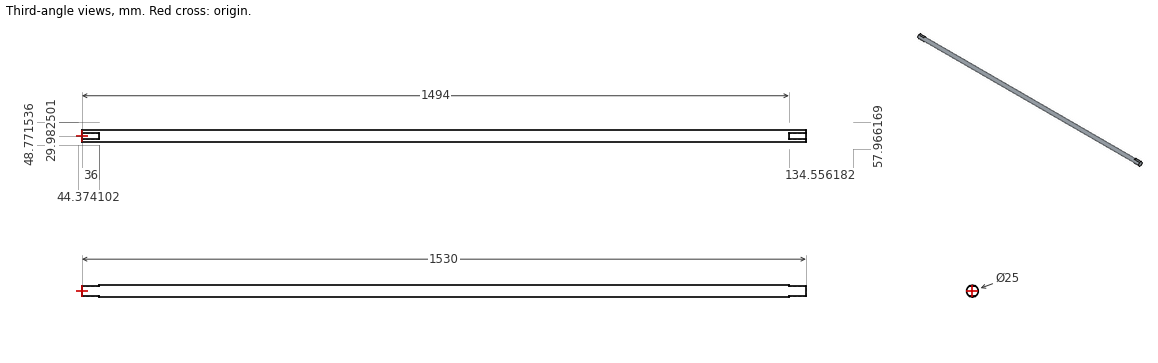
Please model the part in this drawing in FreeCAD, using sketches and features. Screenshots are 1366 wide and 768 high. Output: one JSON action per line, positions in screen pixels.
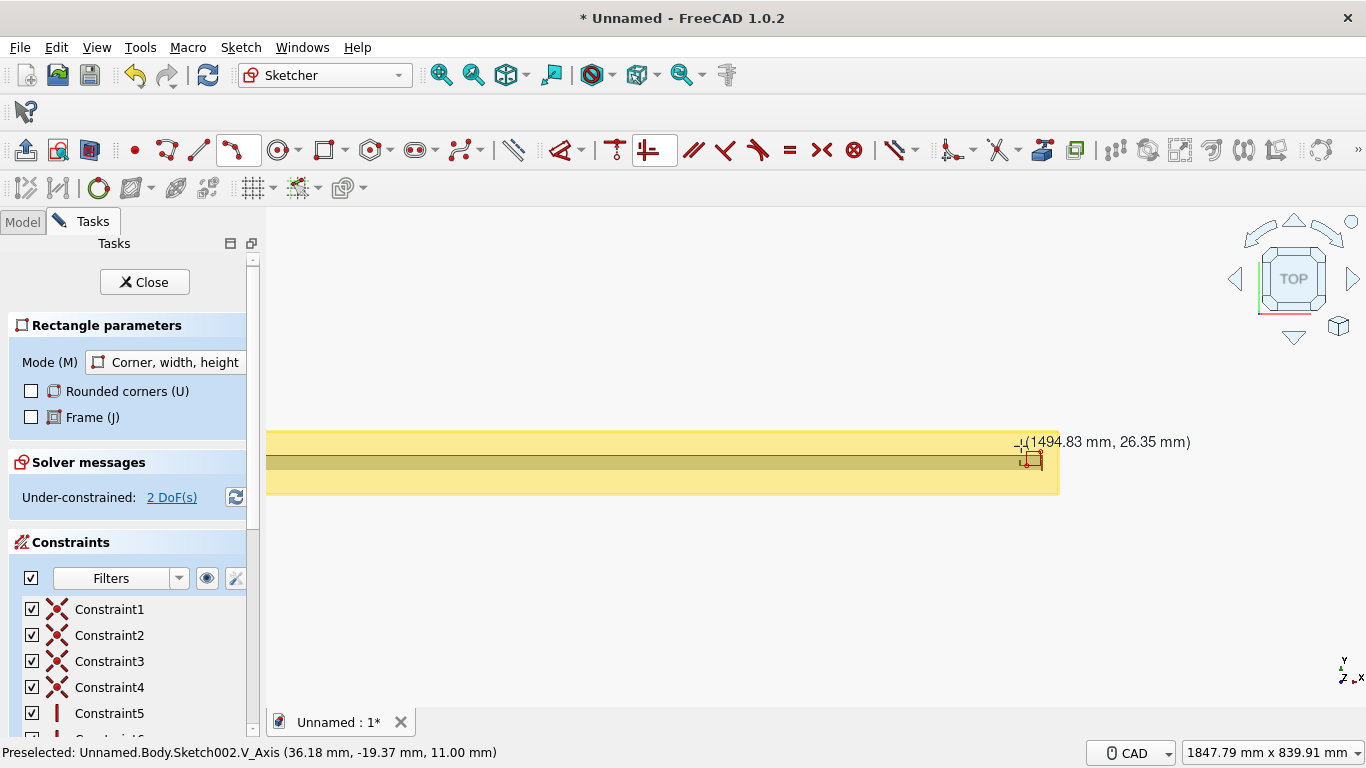
{"action": "left_click", "coordinate": [1020, 445]}
{"action": "mouse_move", "coordinate": [1100, 480]}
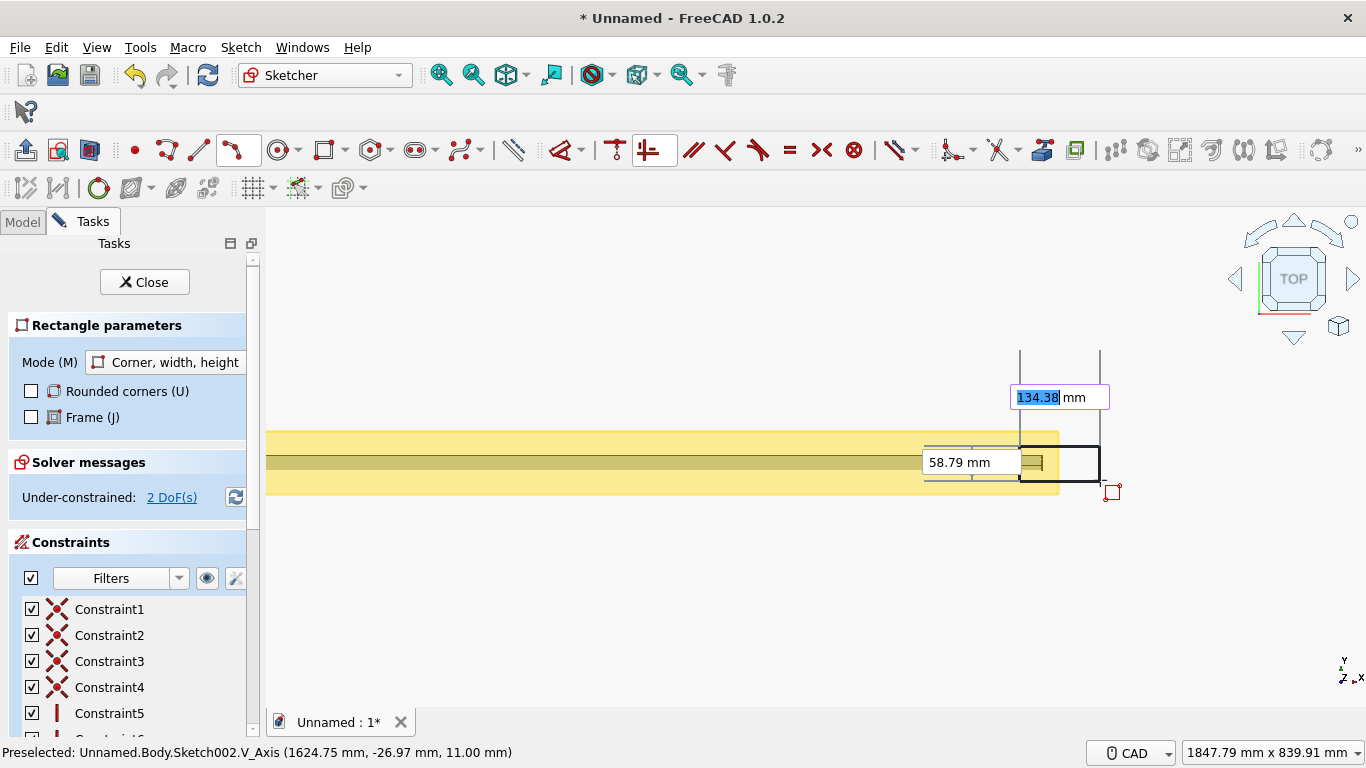
{"action": "type", "text": "134.556182"}
{"action": "key", "text": "Tab"}
{"action": "type", "text": "57.966169"}
{"action": "key", "text": "Return"}
{"action": "key", "text": "Escape"}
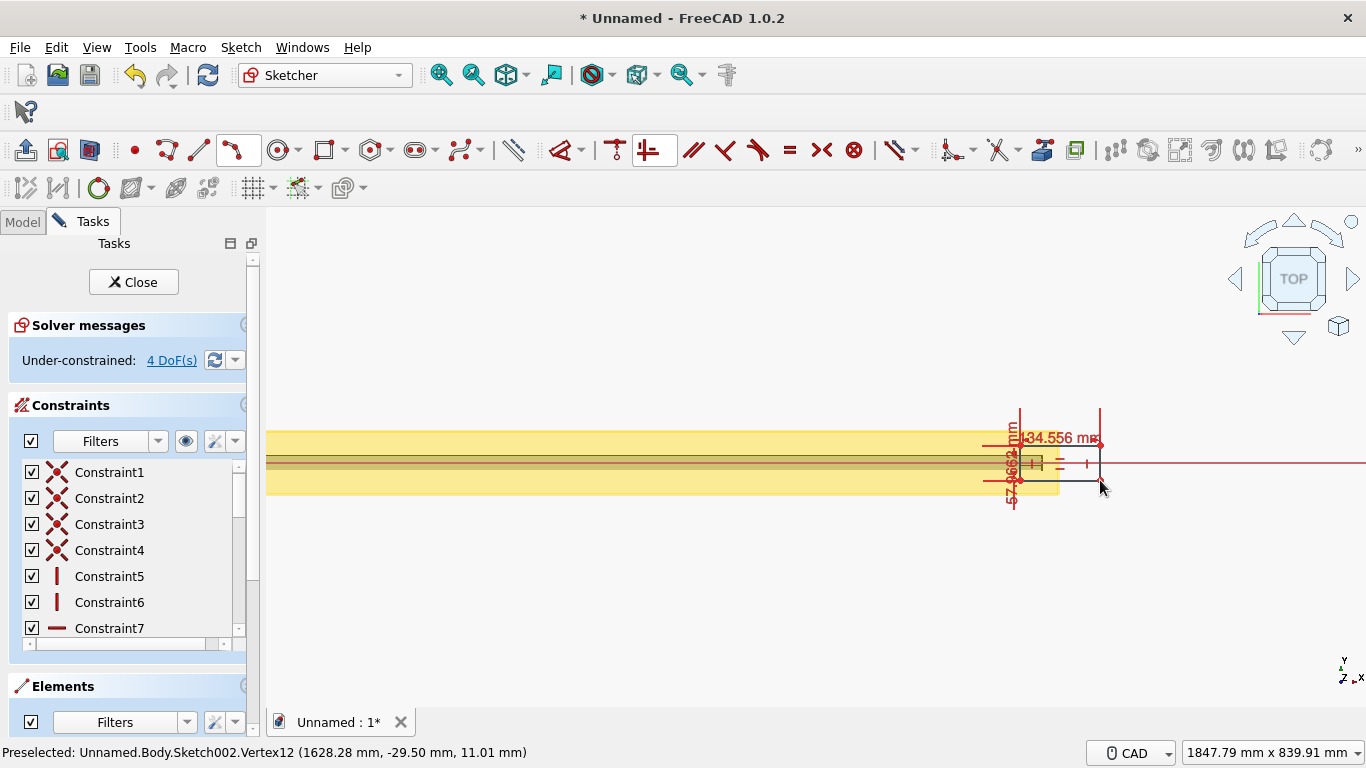
{"action": "left_click", "coordinate": [560, 150]}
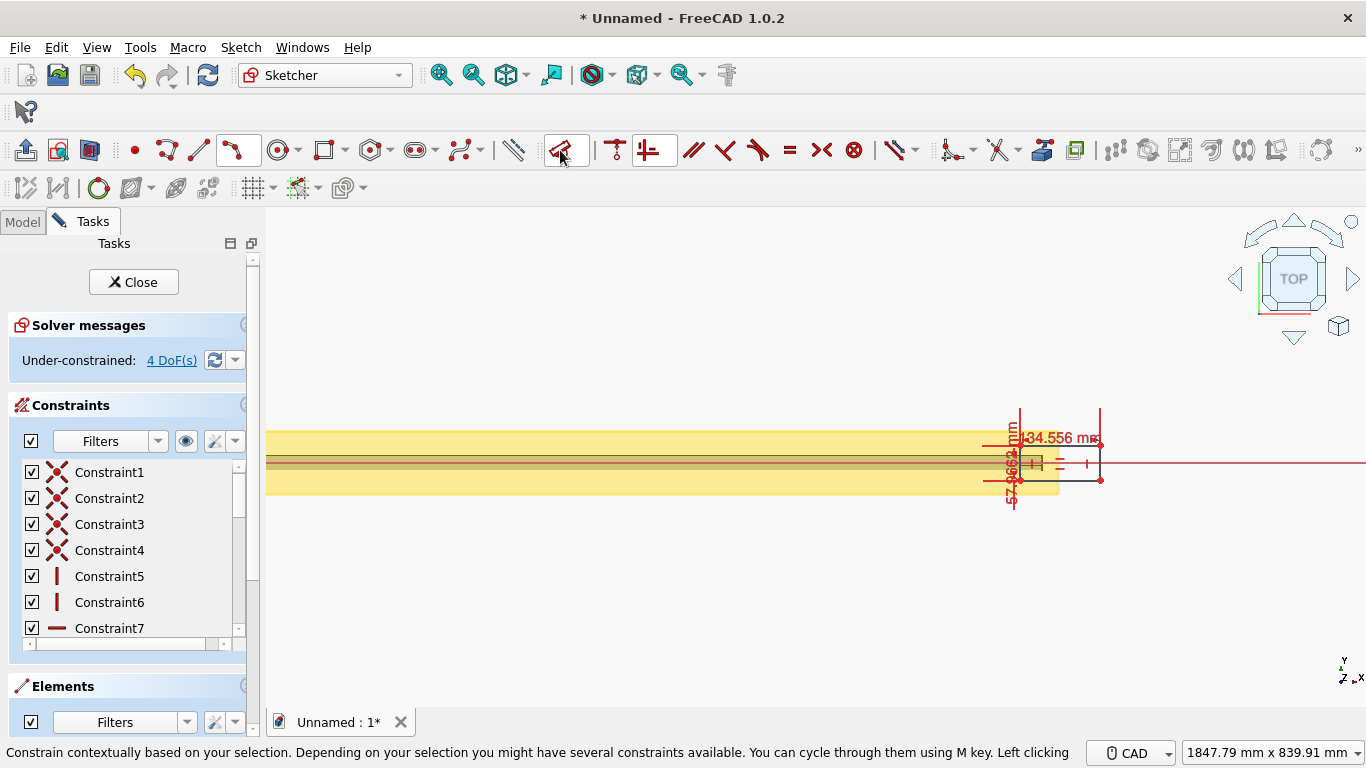
{"action": "scroll", "coordinate": [1021, 446], "scroll_direction": "down", "scroll_amount": 2}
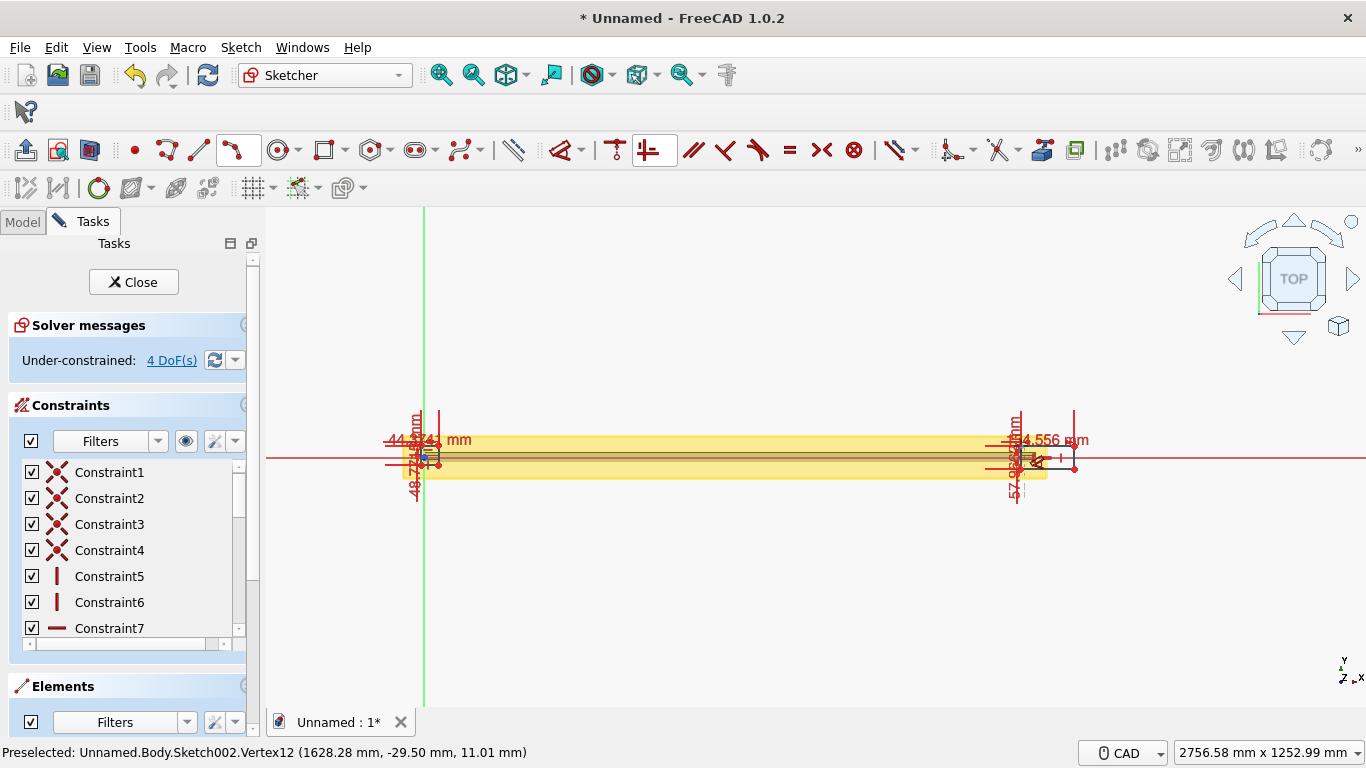
{"action": "scroll", "coordinate": [439, 465], "scroll_direction": "up", "scroll_amount": 6}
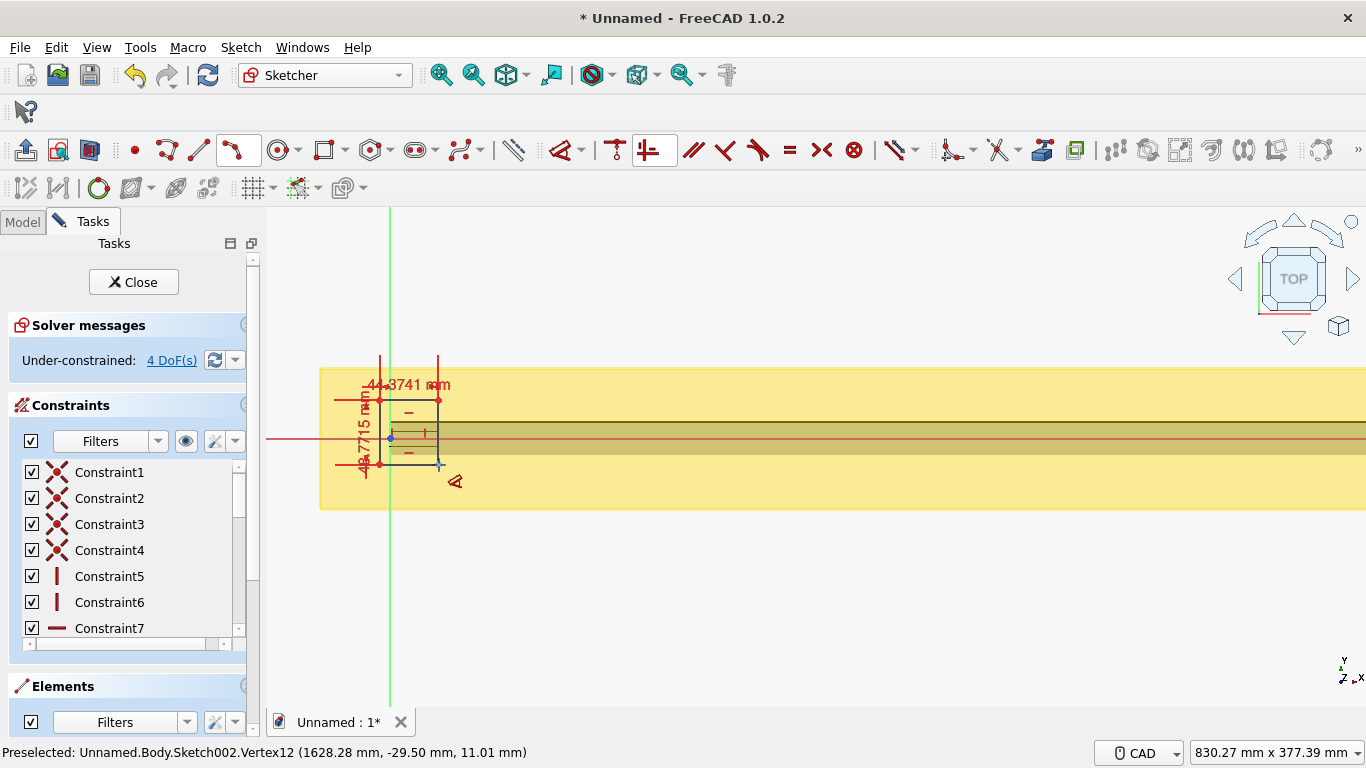
{"action": "left_click", "coordinate": [438, 465]}
{"action": "left_click", "coordinate": [414, 499]}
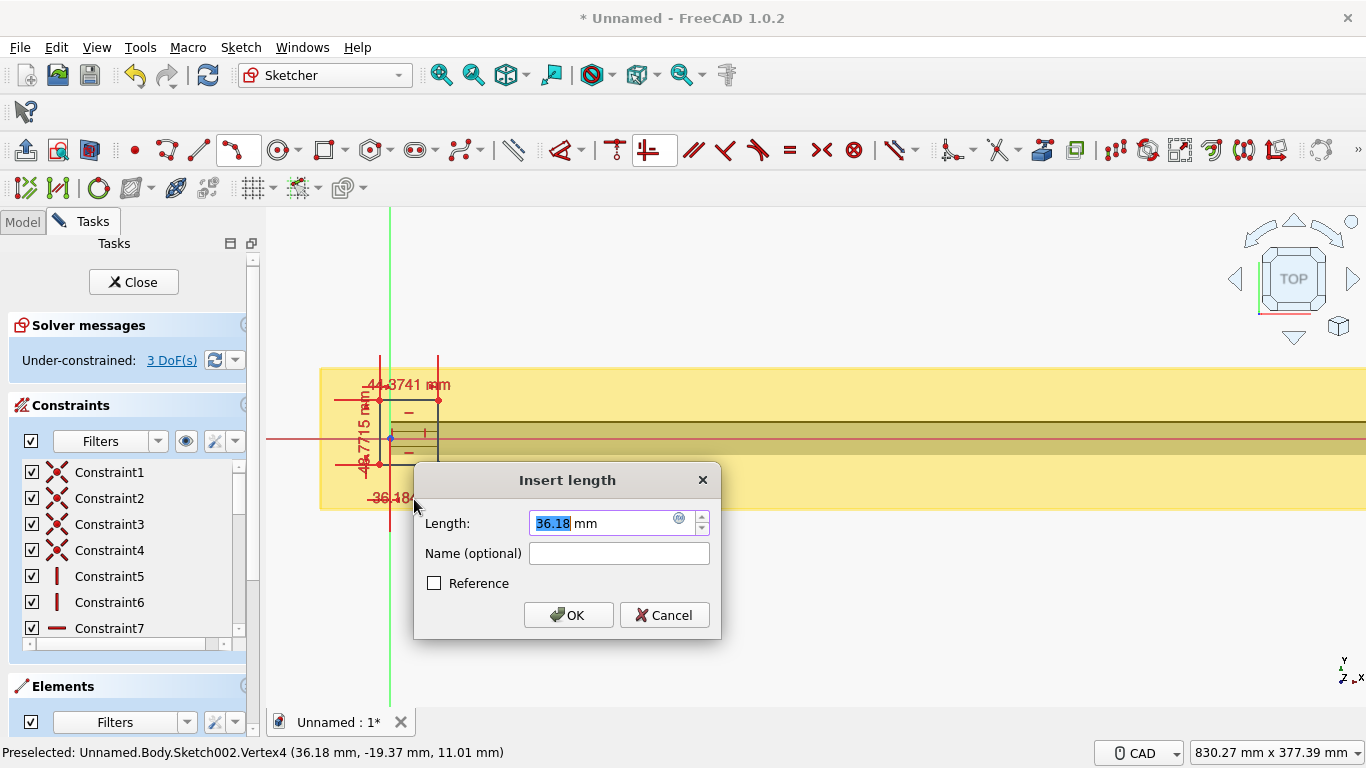
{"action": "type", "text": "36"}
{"action": "key", "text": "Return"}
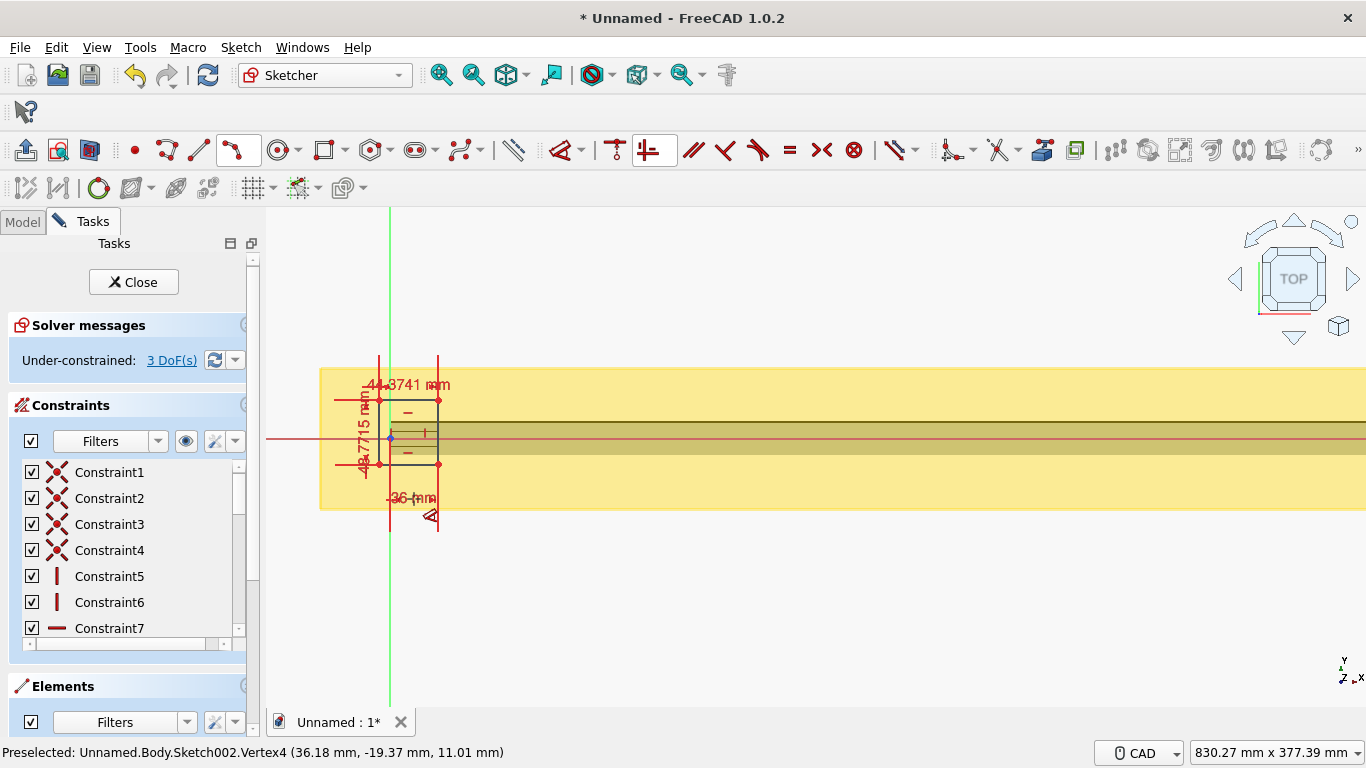
{"action": "scroll", "coordinate": [439, 465], "scroll_direction": "down", "scroll_amount": 6}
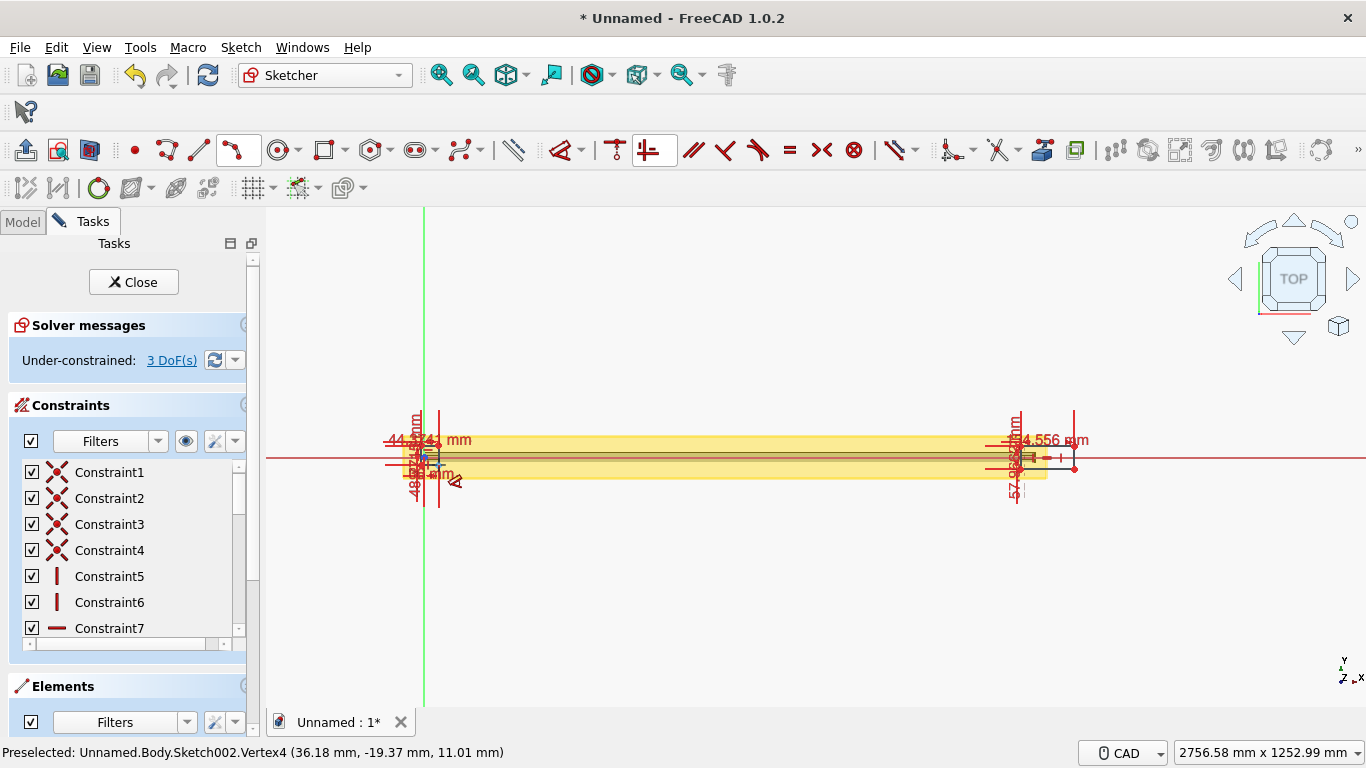
{"action": "left_click", "coordinate": [1021, 446]}
{"action": "left_click", "coordinate": [723, 412]}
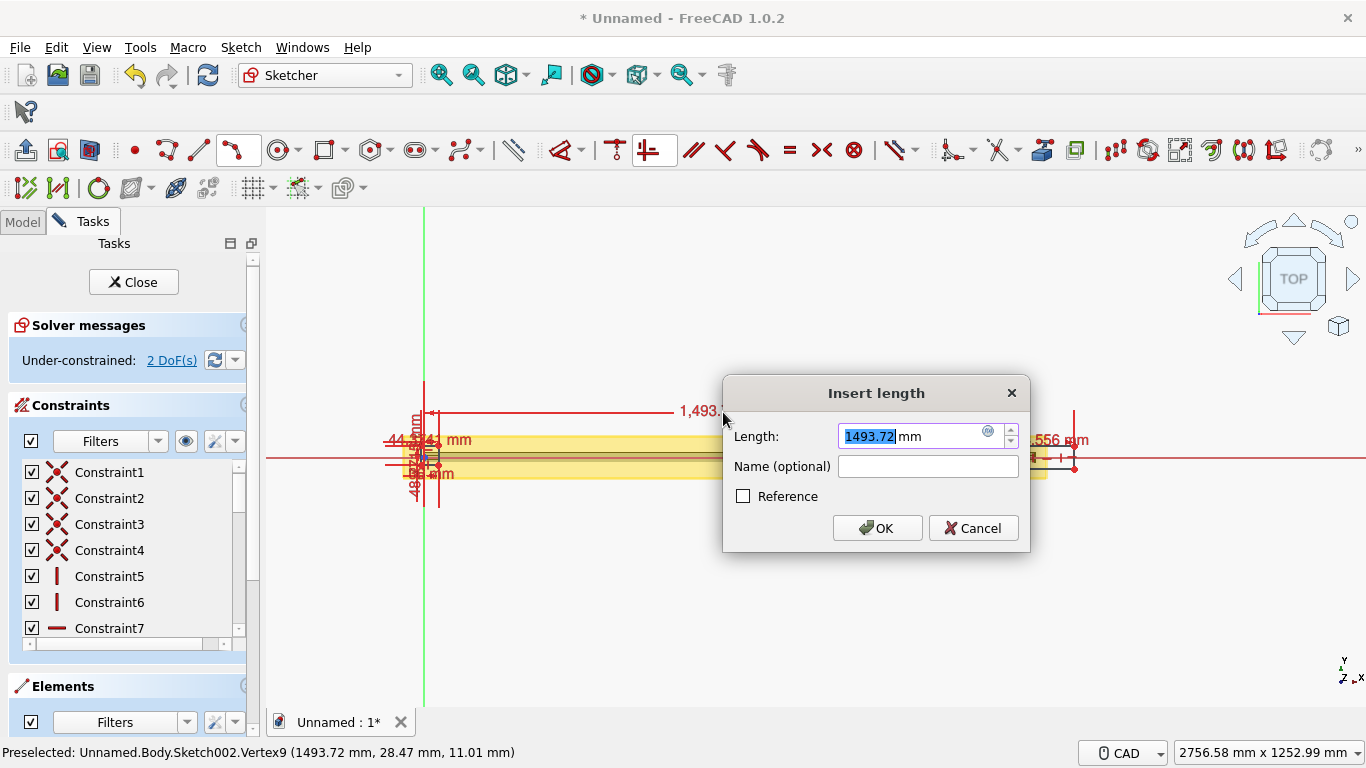
{"action": "type", "text": "1494"}
{"action": "key", "text": "Return"}